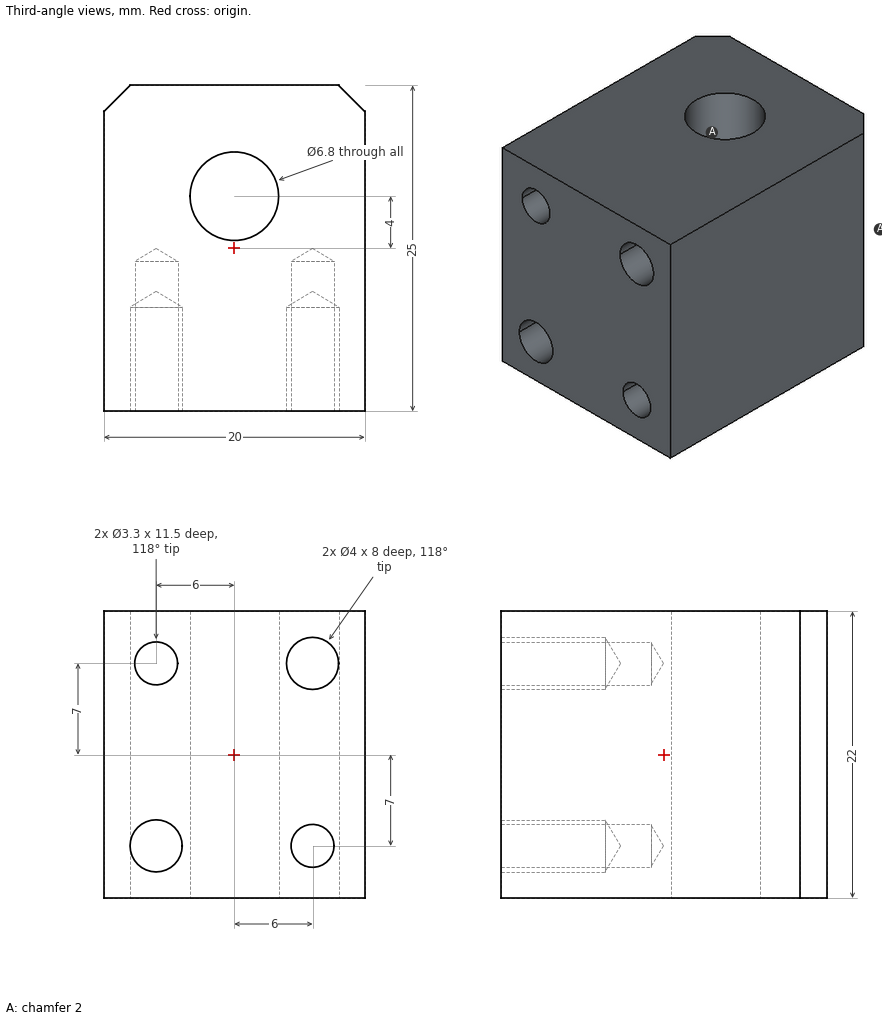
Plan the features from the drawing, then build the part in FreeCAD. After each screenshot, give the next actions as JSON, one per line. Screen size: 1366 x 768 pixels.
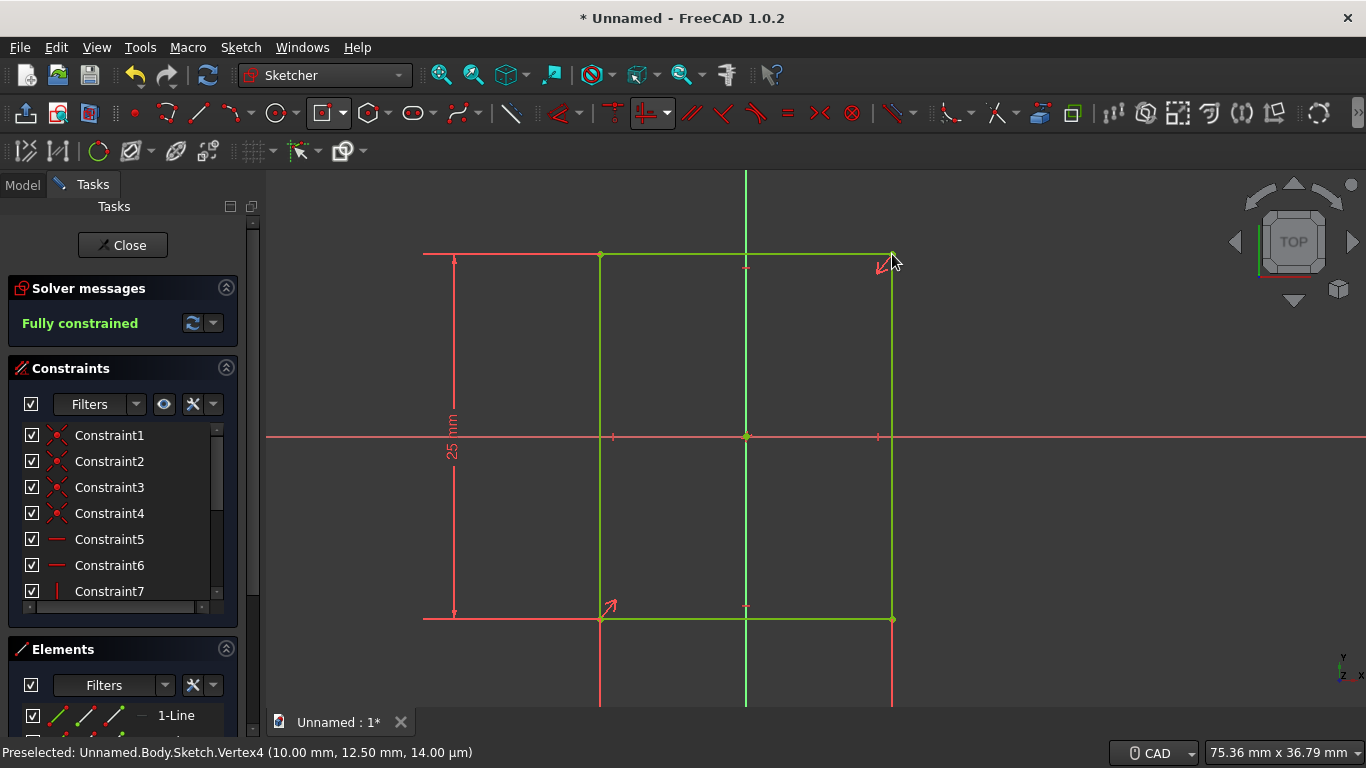
{"action": "left_click", "coordinate": [123, 245]}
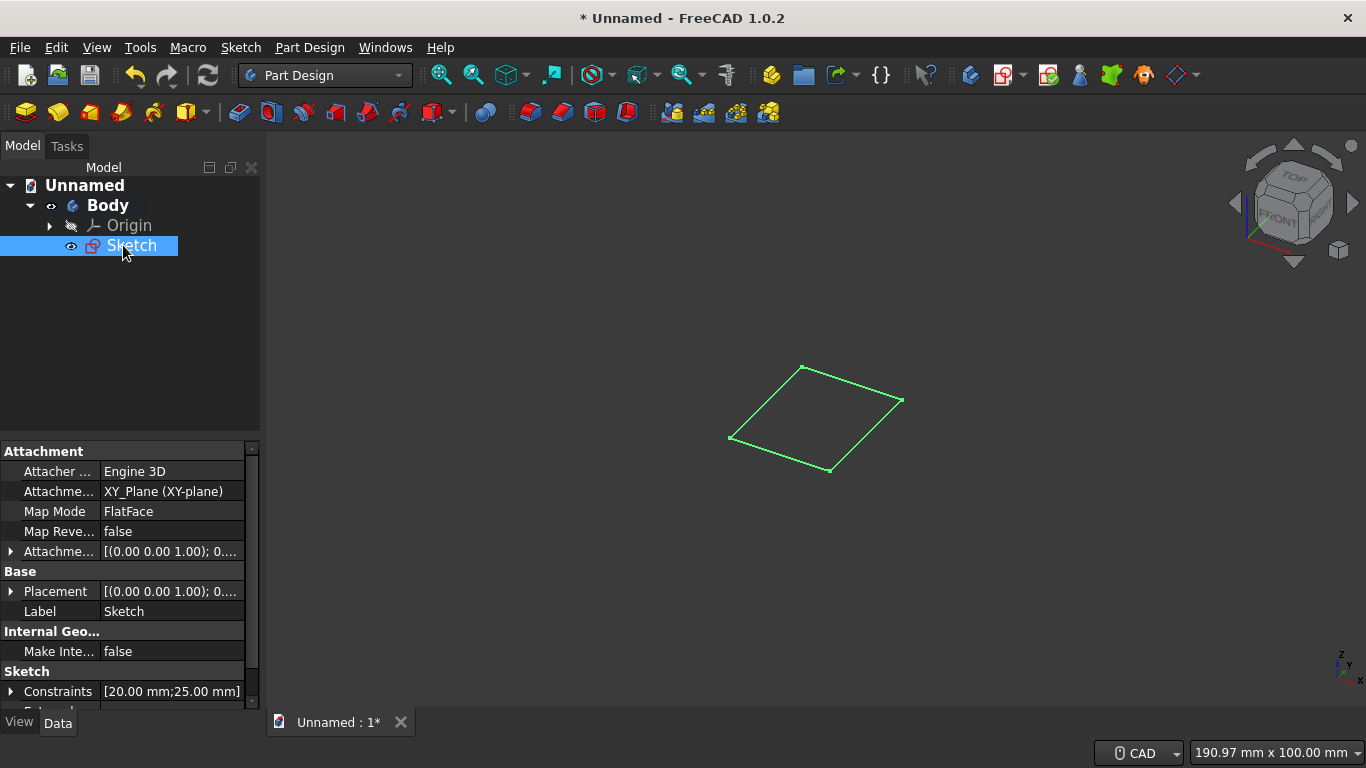
{"action": "left_click", "coordinate": [26, 112]}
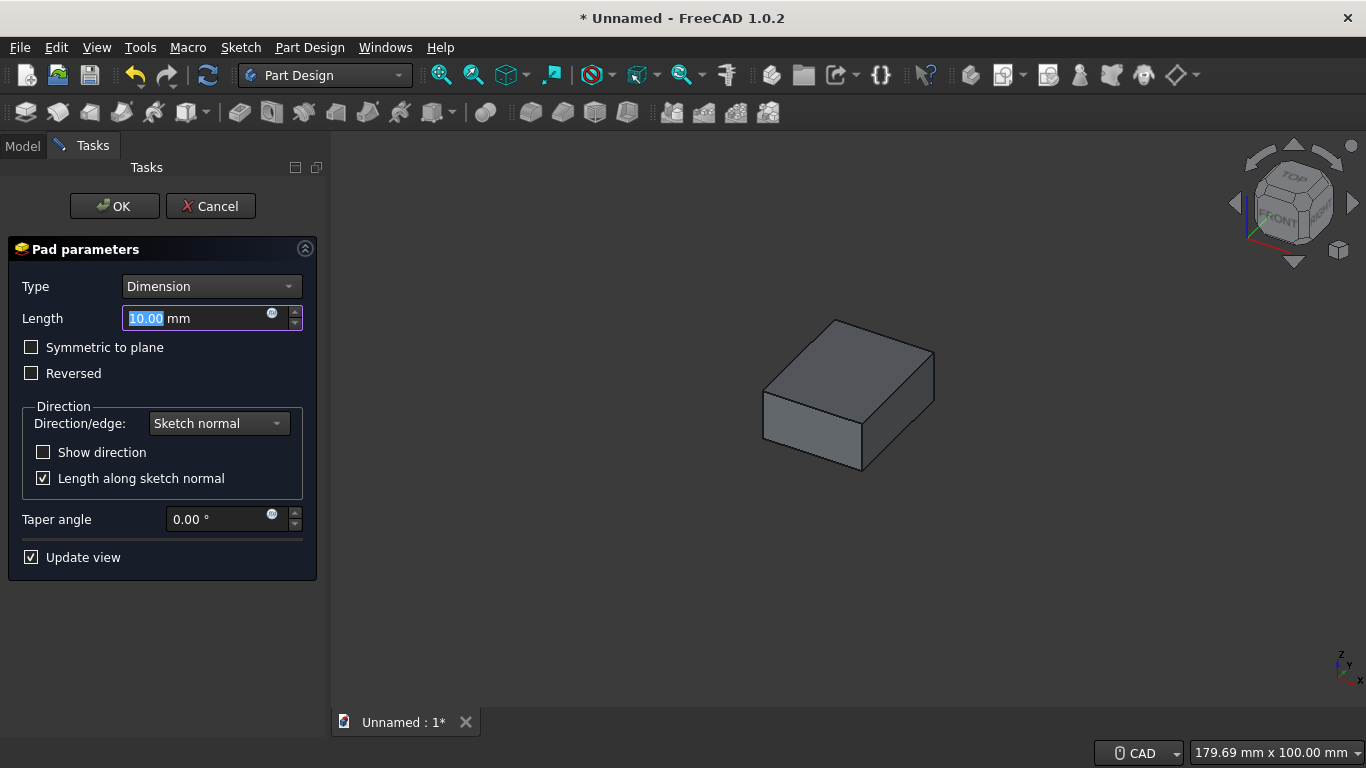
{"action": "type", "text": "22"}
{"action": "key", "text": "Tab"}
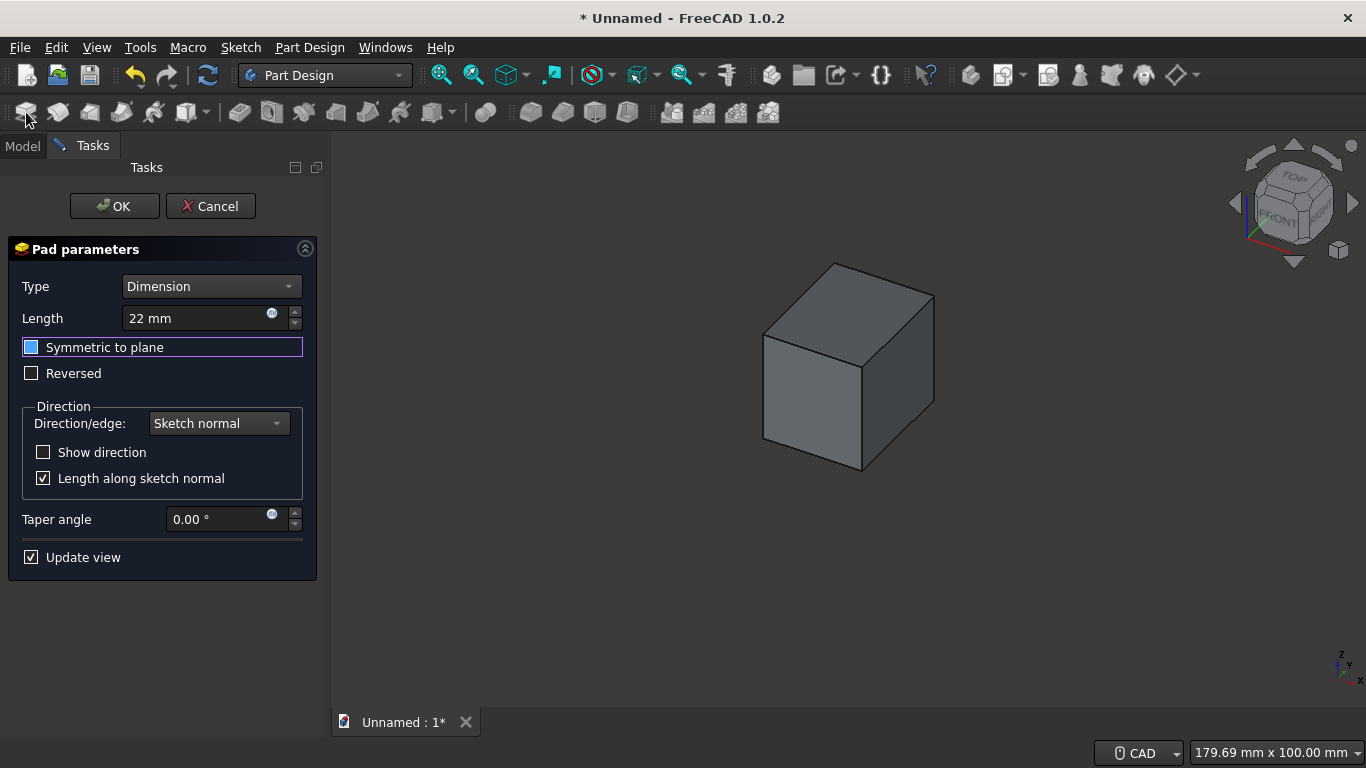
{"action": "left_click", "coordinate": [30, 347]}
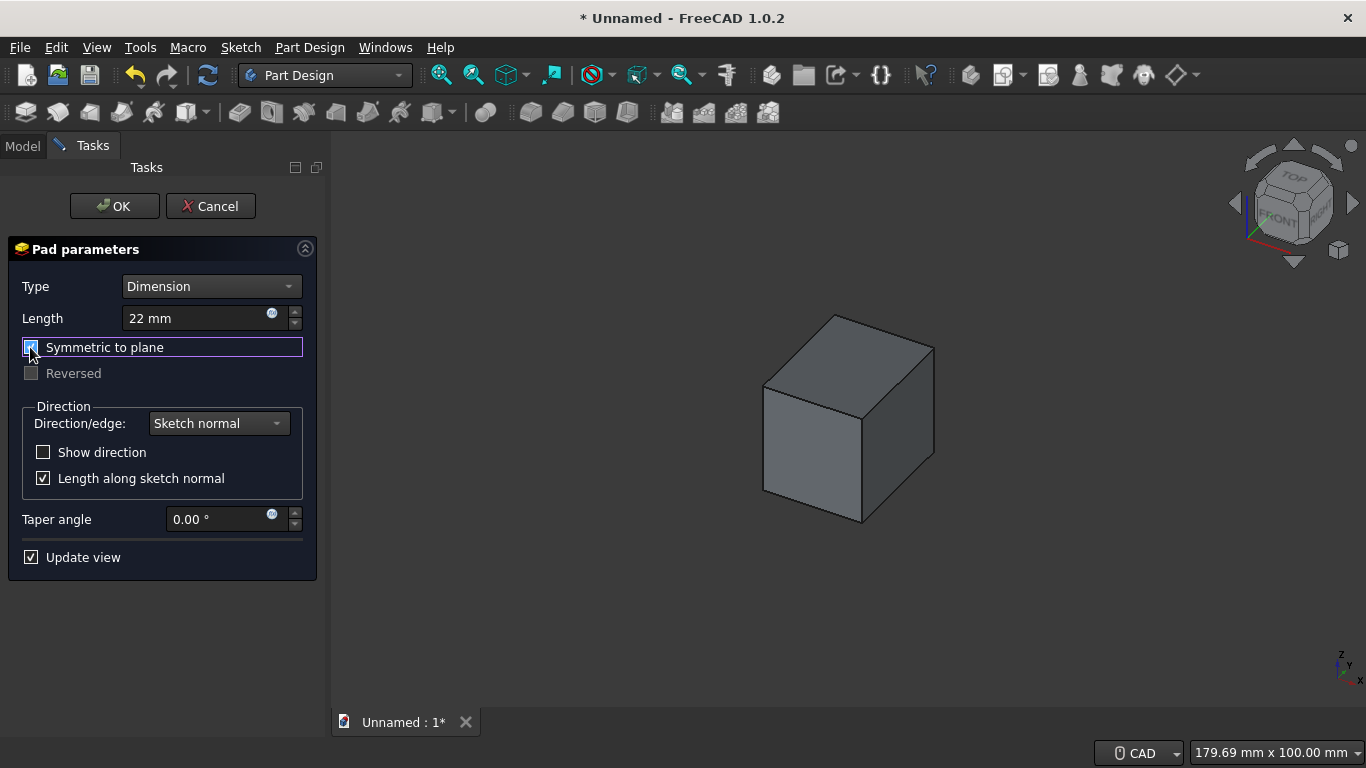
{"action": "left_click", "coordinate": [115, 206]}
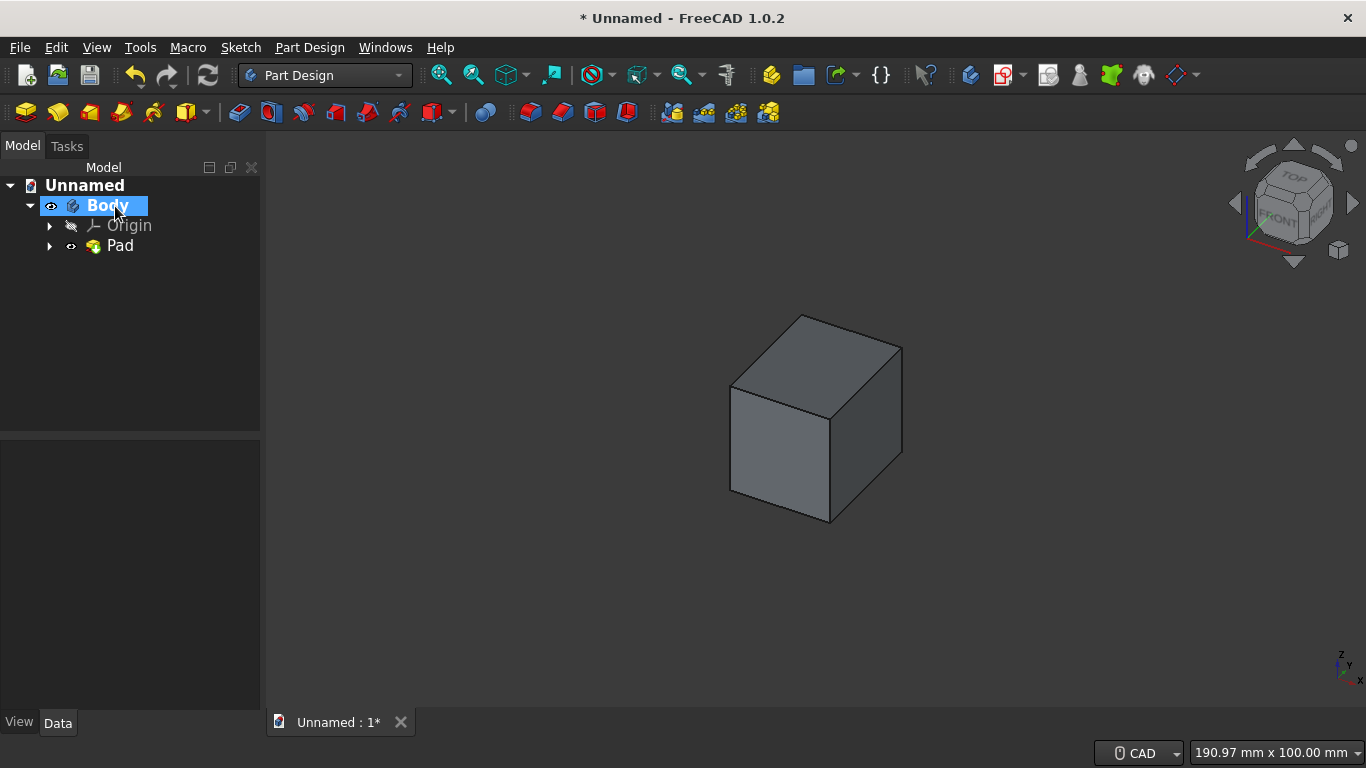
{"action": "left_click", "coordinate": [442, 76]}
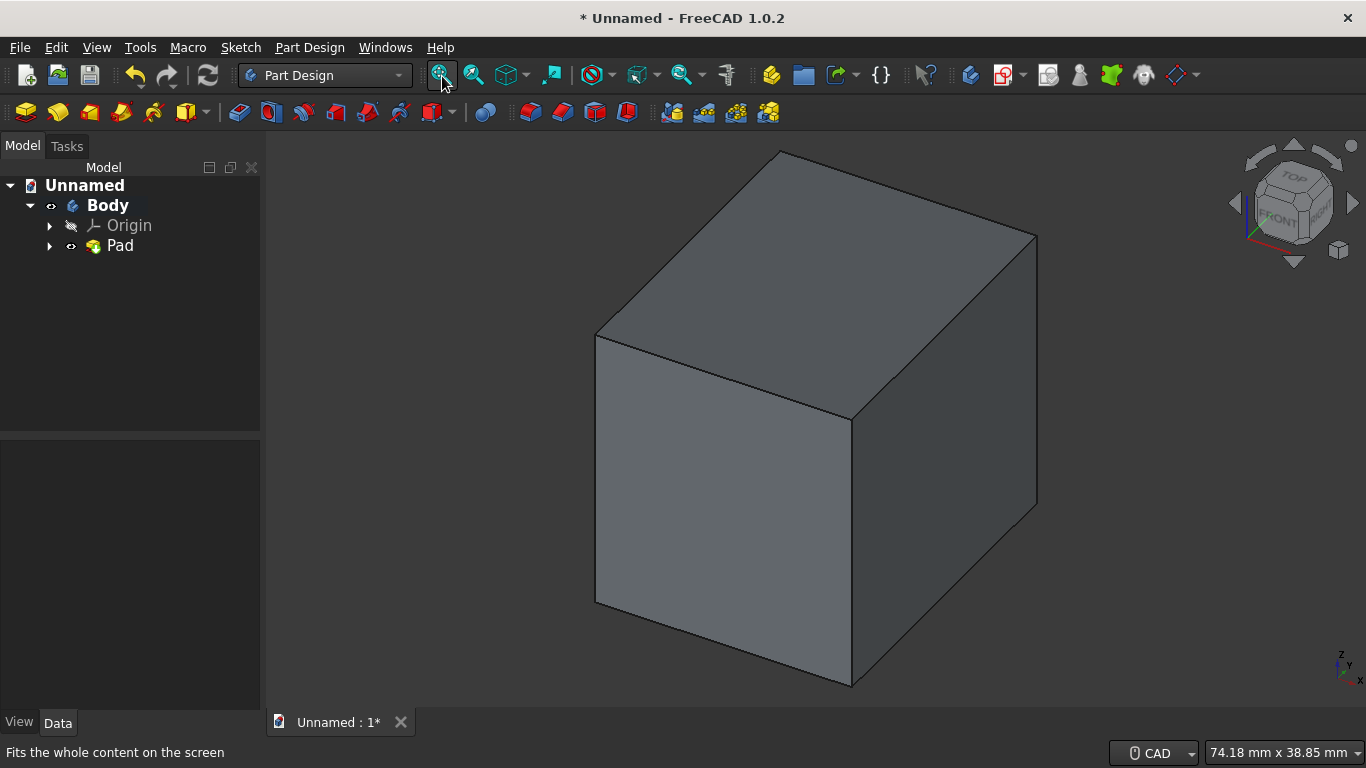
{"action": "key", "text": "0"}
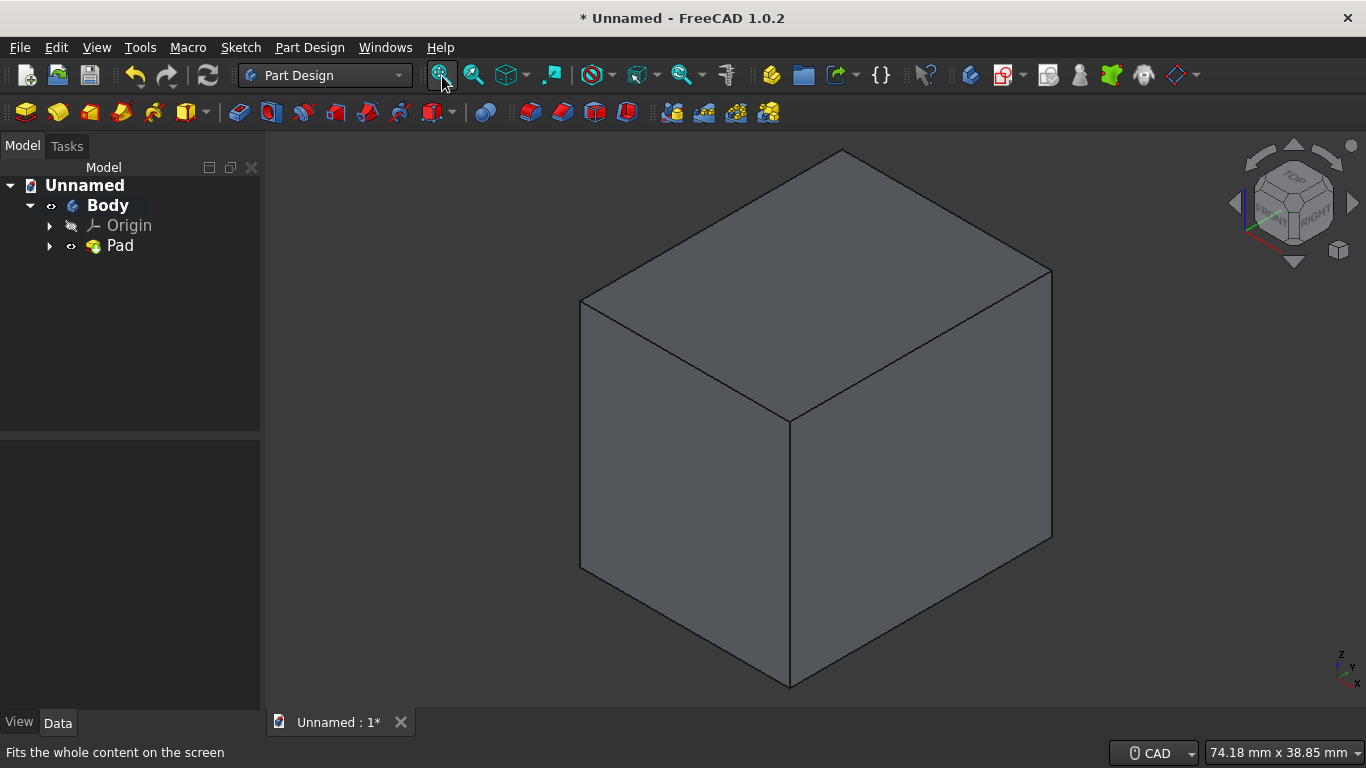
{"action": "key", "text": "2"}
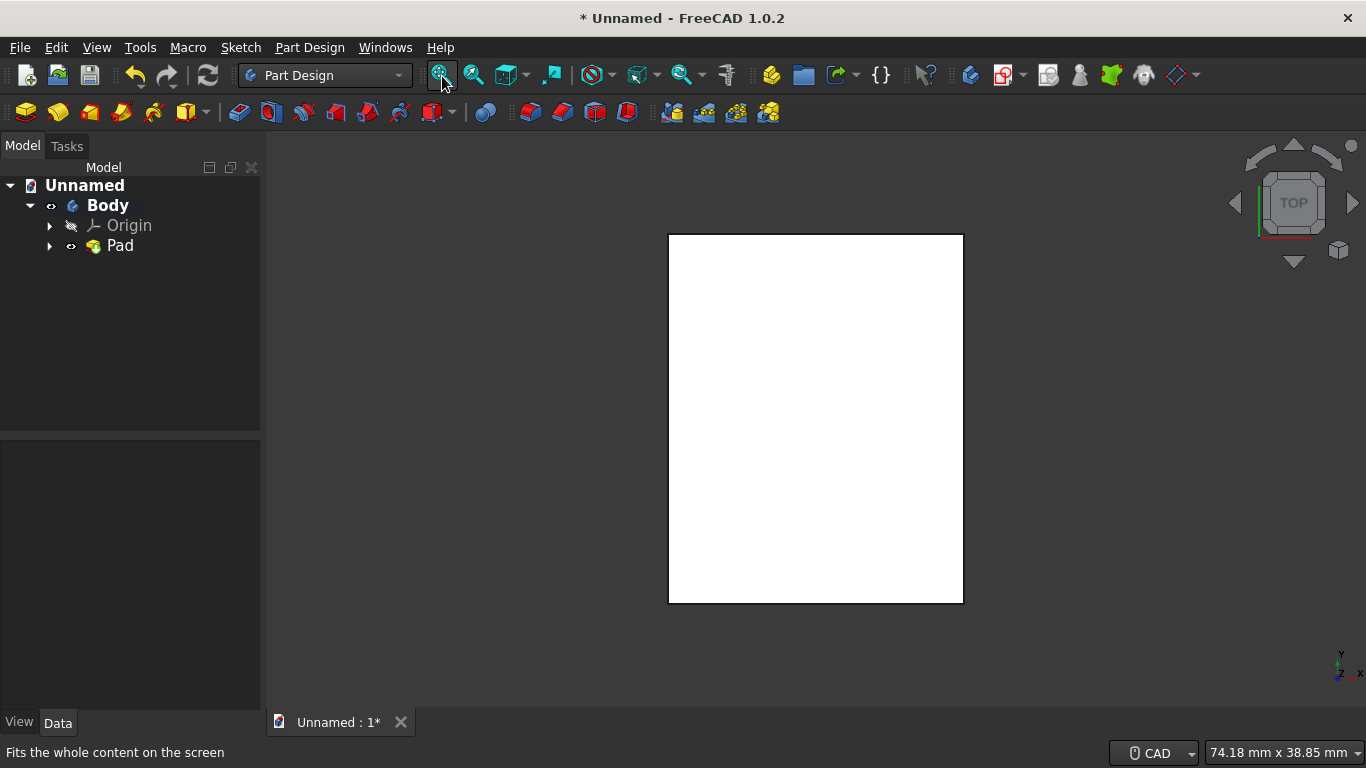
{"action": "key", "text": "1"}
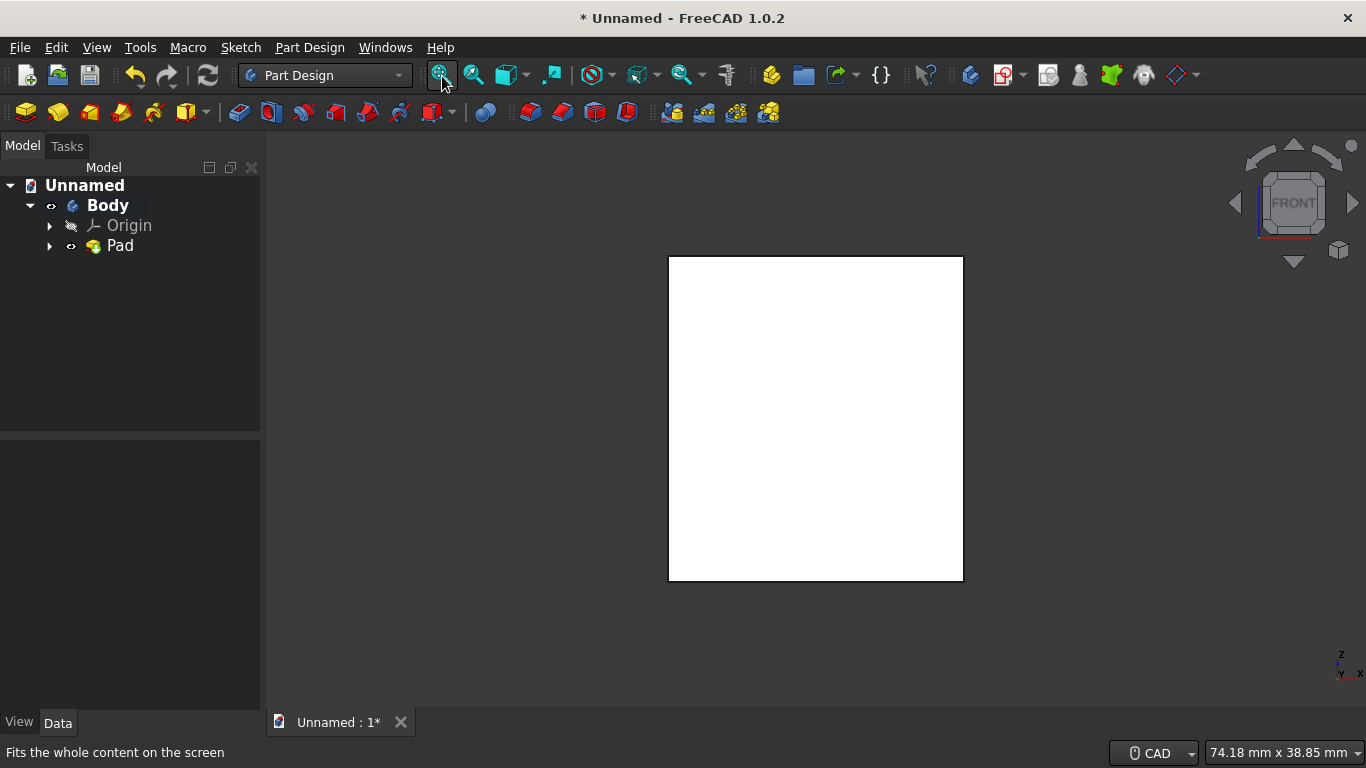
{"action": "key", "text": "3"}